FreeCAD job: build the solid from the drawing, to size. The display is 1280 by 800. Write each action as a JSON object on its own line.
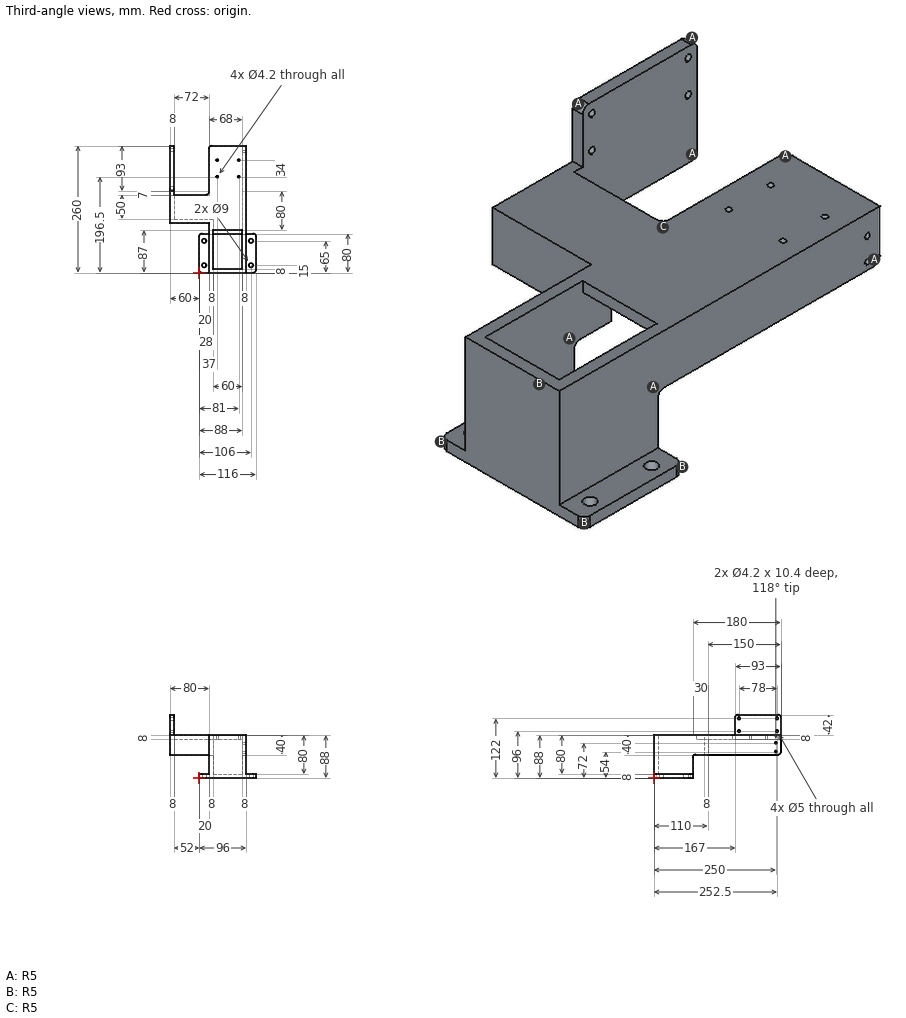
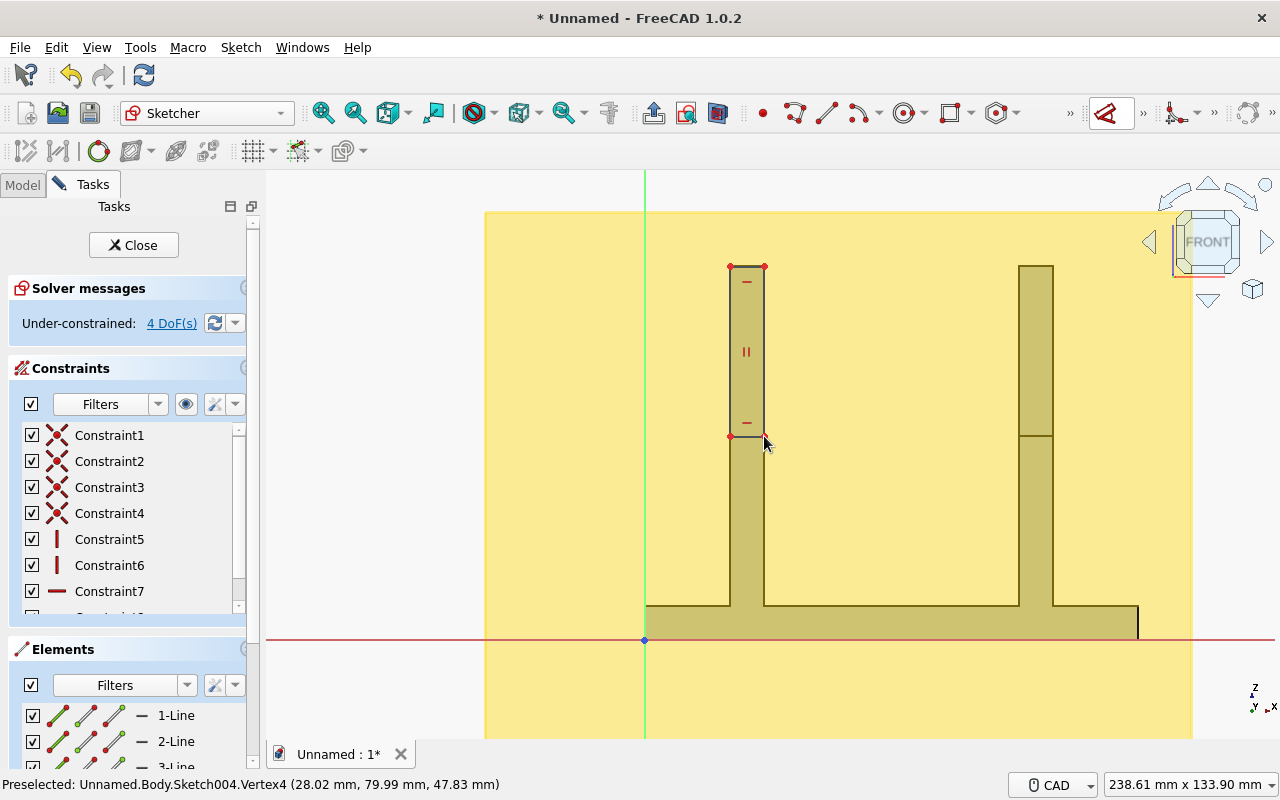
{"action": "scroll", "coordinate": [740, 437], "scroll_direction": "up", "scroll_amount": 2}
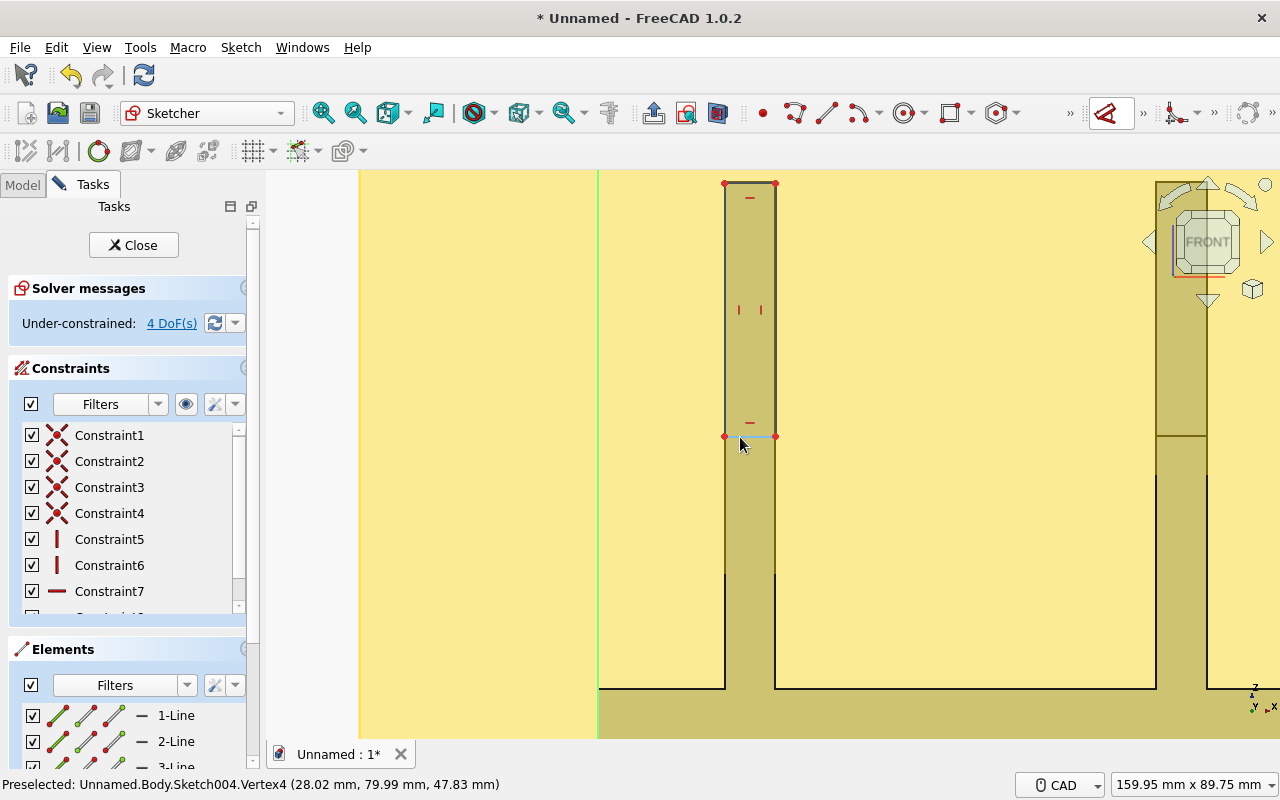
{"action": "left_click", "coordinate": [740, 437]}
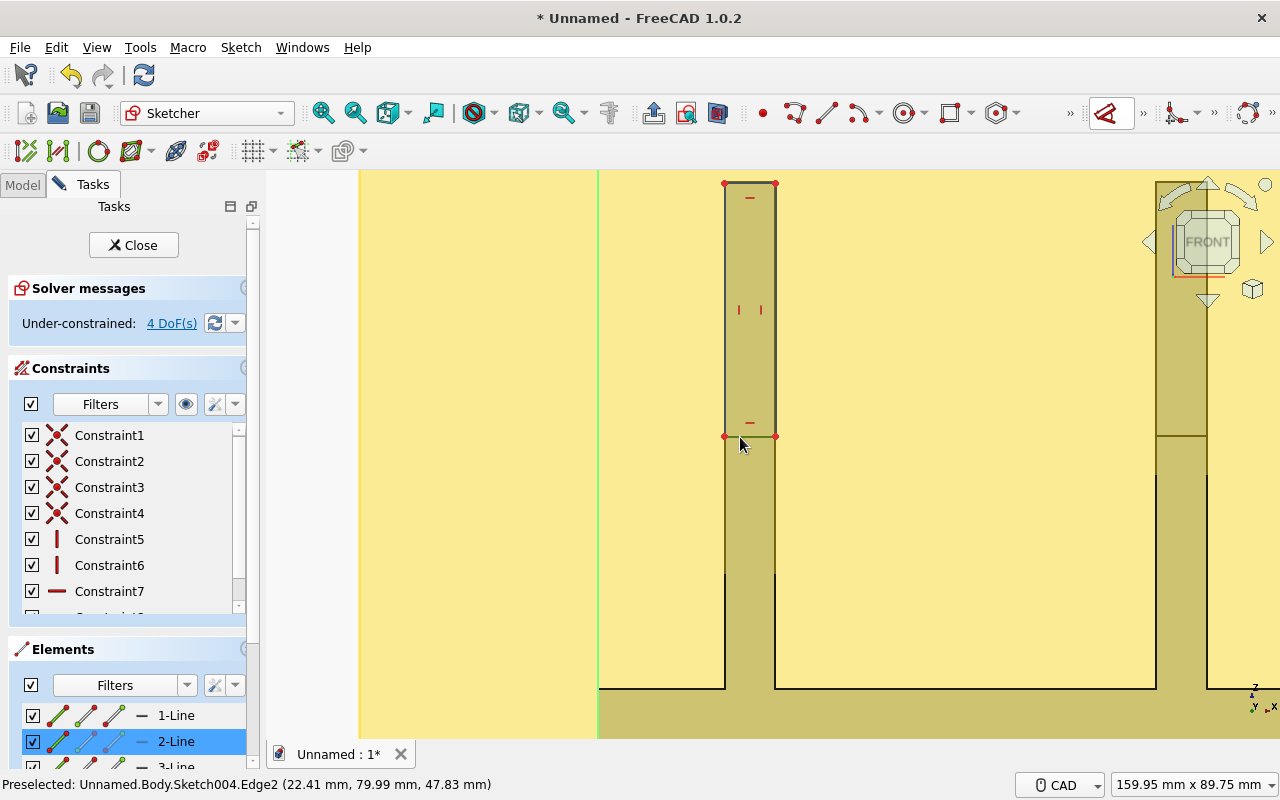
{"action": "key", "text": "l"}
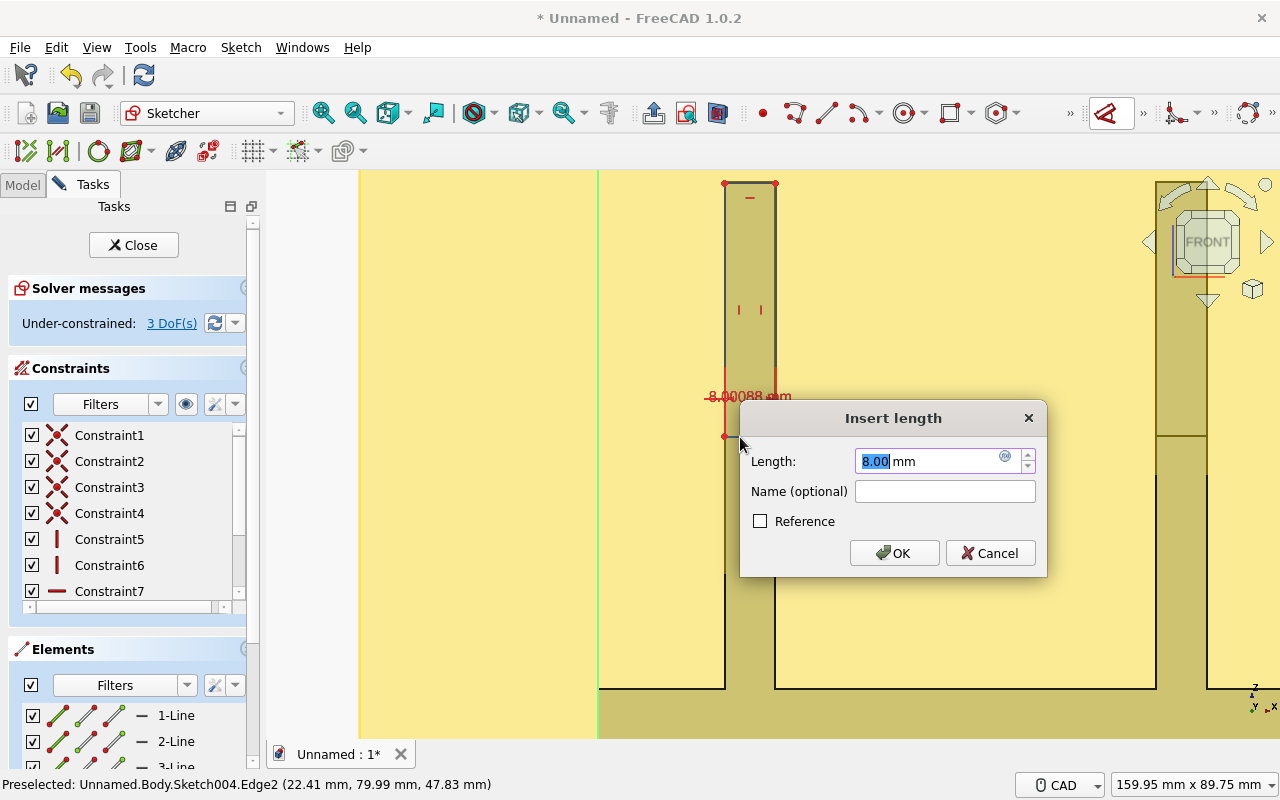
{"action": "type", "text": "8"}
{"action": "key", "text": "Return"}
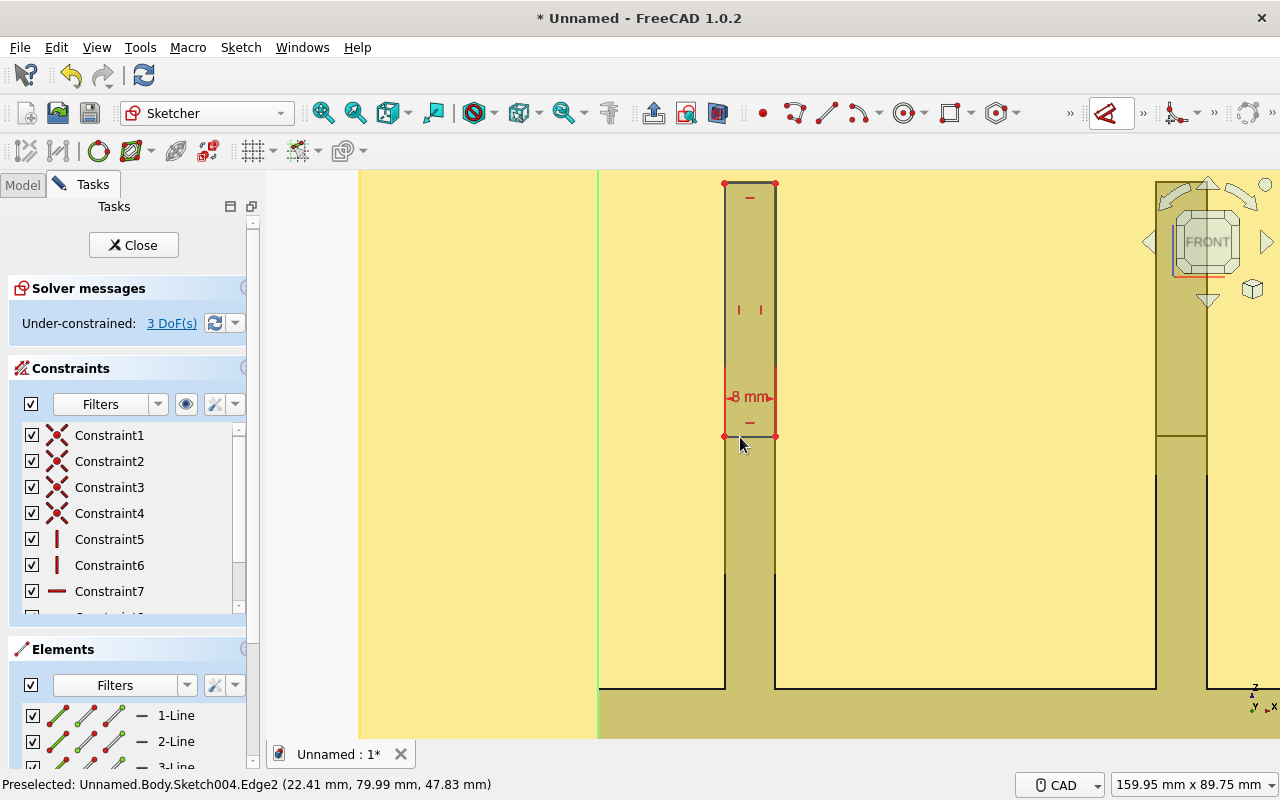
{"action": "left_click", "coordinate": [725, 259]}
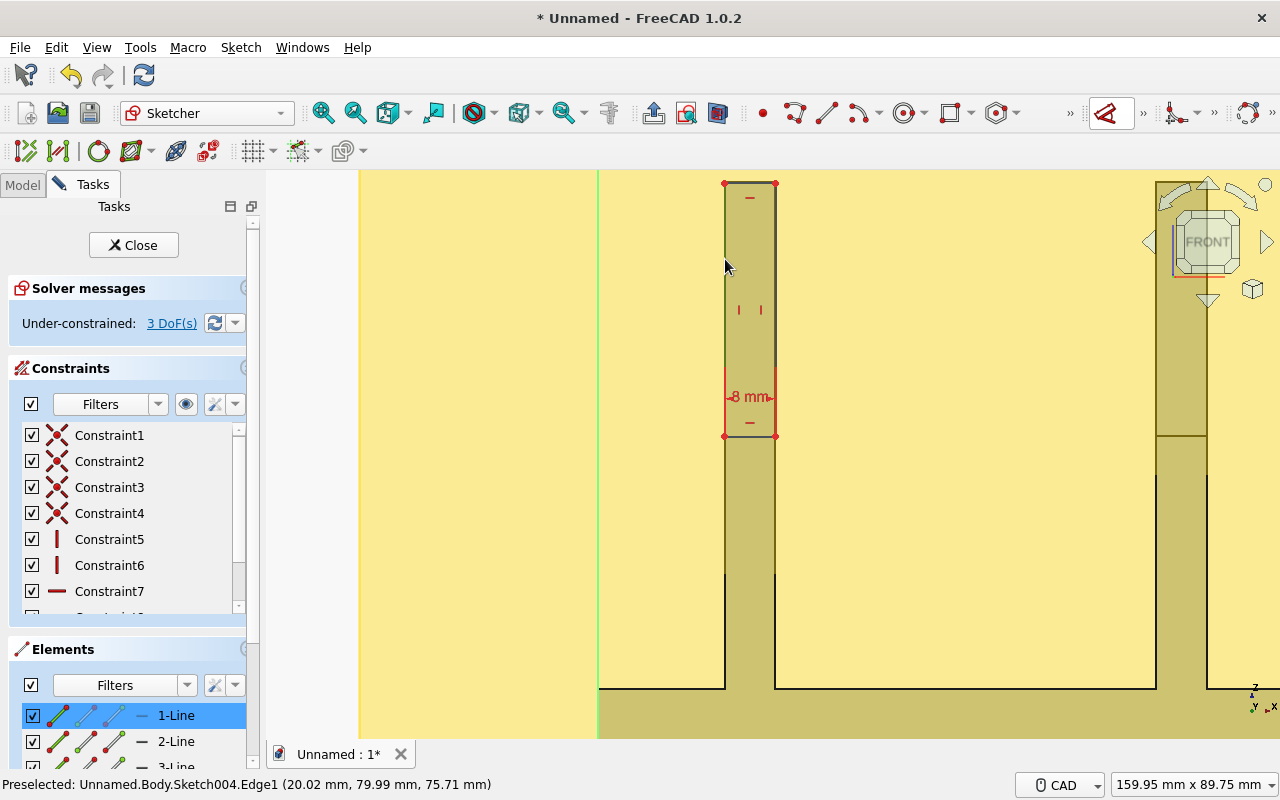
{"action": "left_click", "coordinate": [1128, 114]}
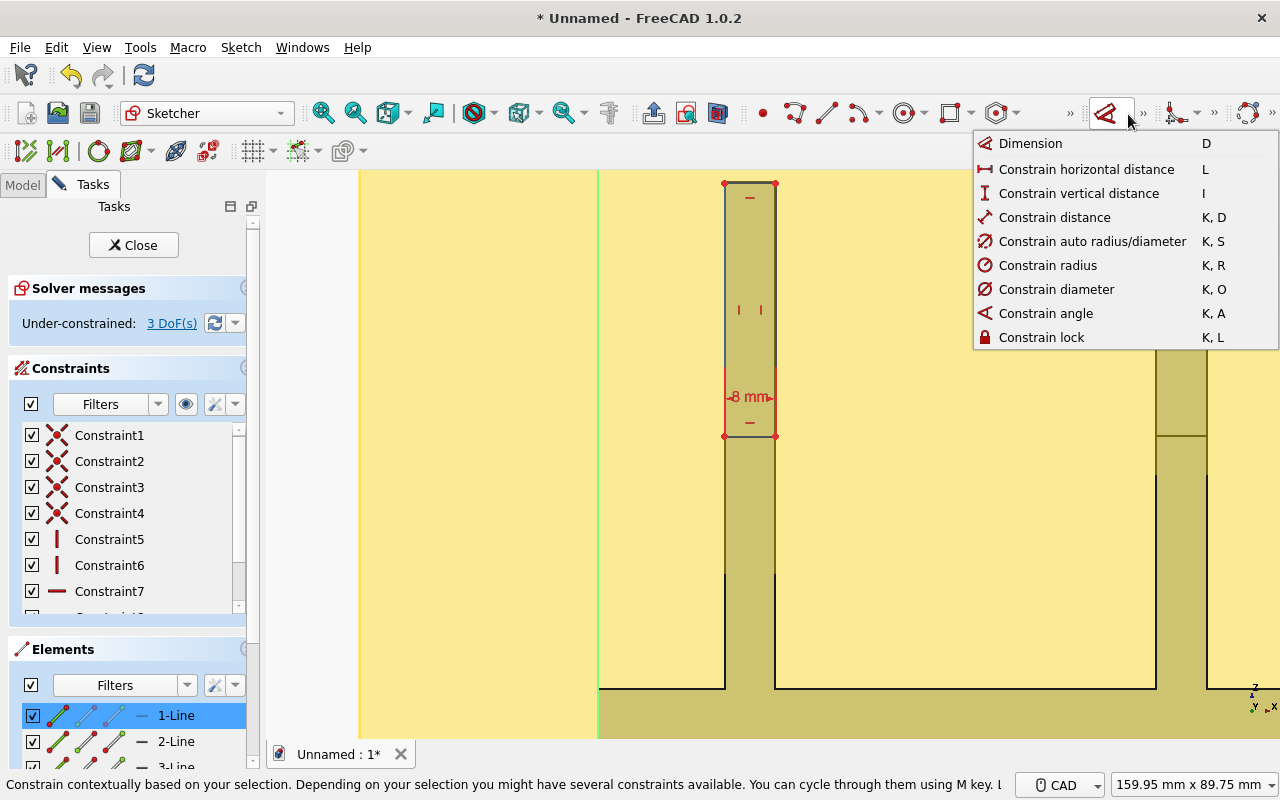
{"action": "left_click", "coordinate": [1126, 193]}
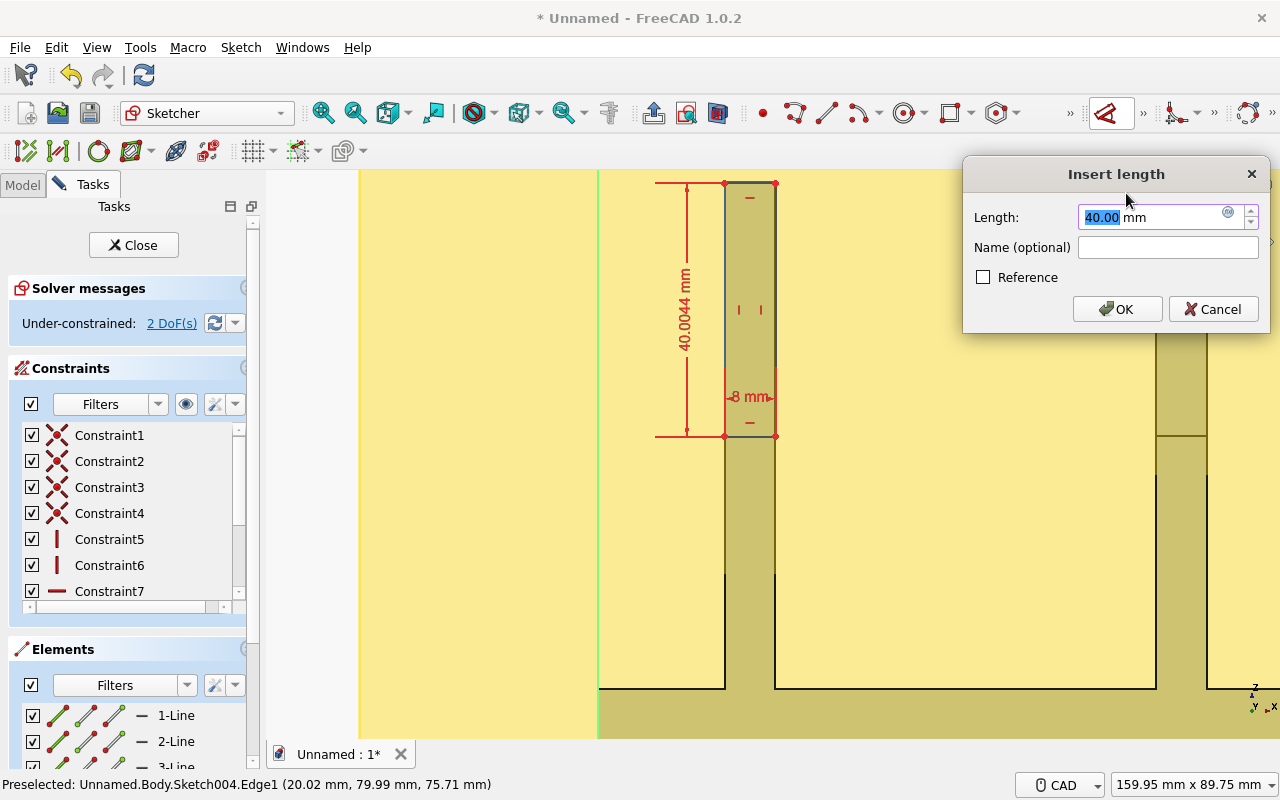
{"action": "type", "text": "40"}
{"action": "key", "text": "Return"}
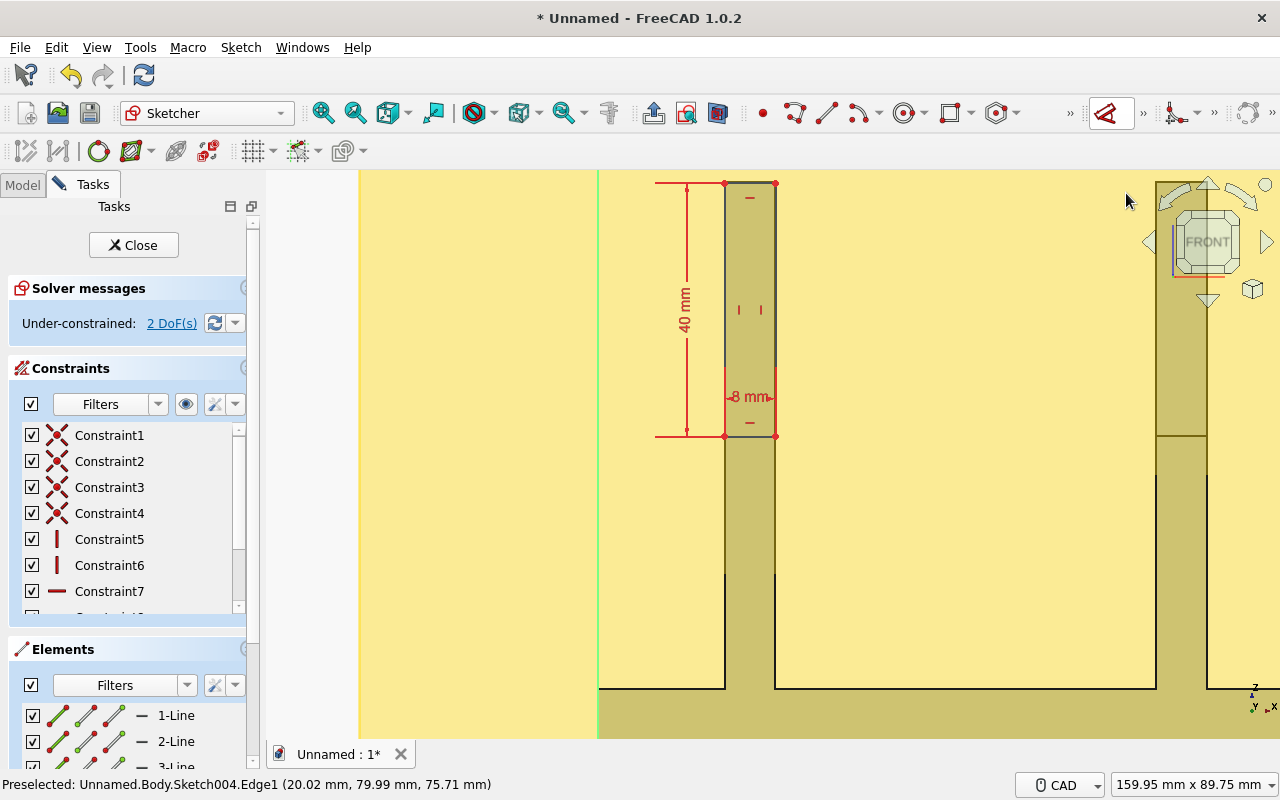
{"action": "scroll", "coordinate": [741, 441], "scroll_direction": "down", "scroll_amount": 2}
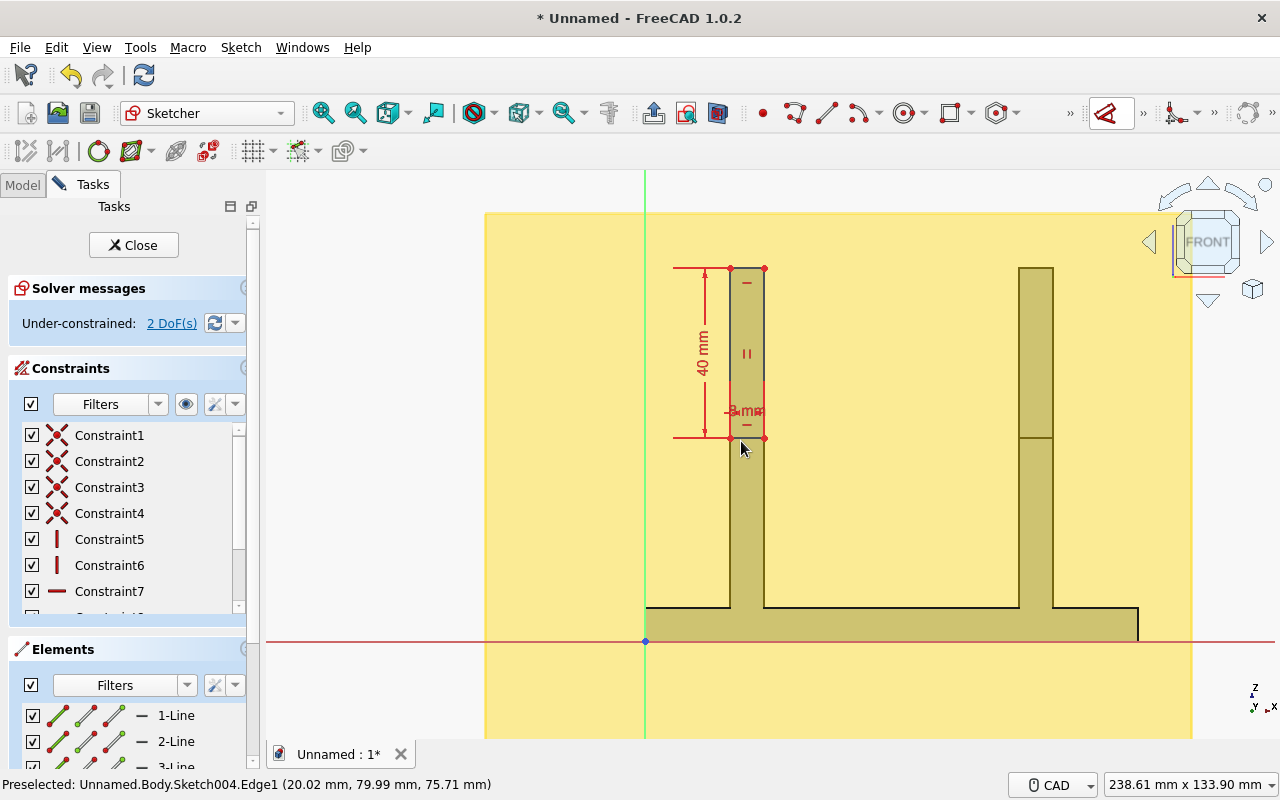
{"action": "left_click", "coordinate": [730, 268]}